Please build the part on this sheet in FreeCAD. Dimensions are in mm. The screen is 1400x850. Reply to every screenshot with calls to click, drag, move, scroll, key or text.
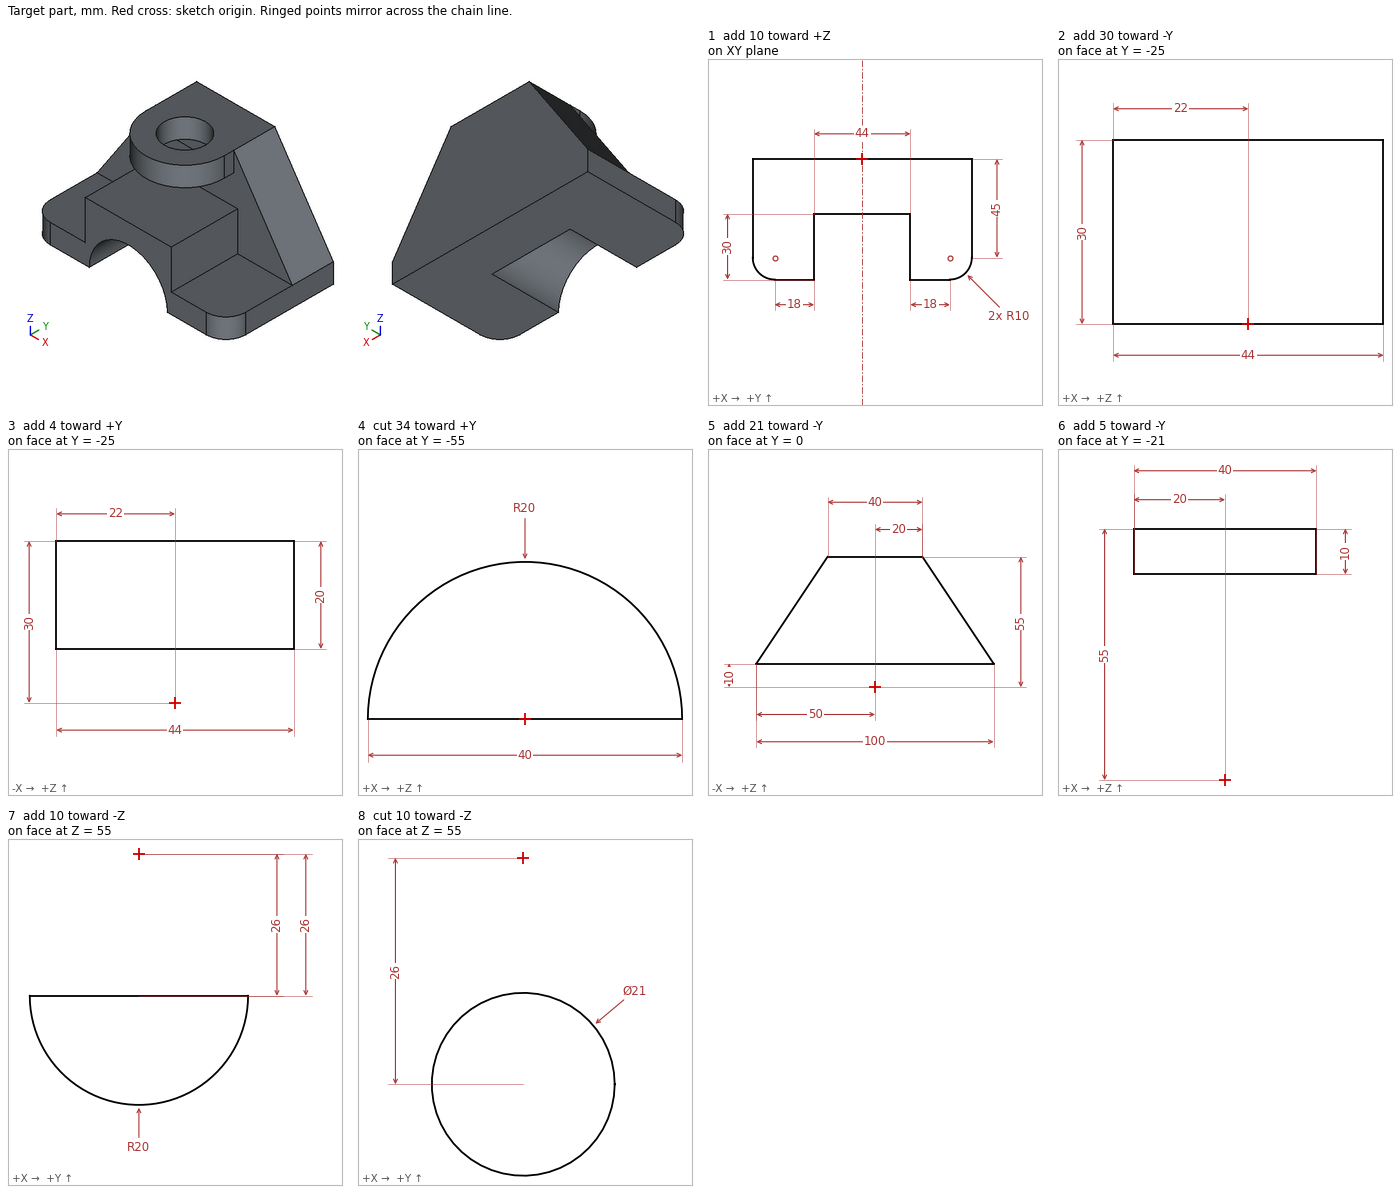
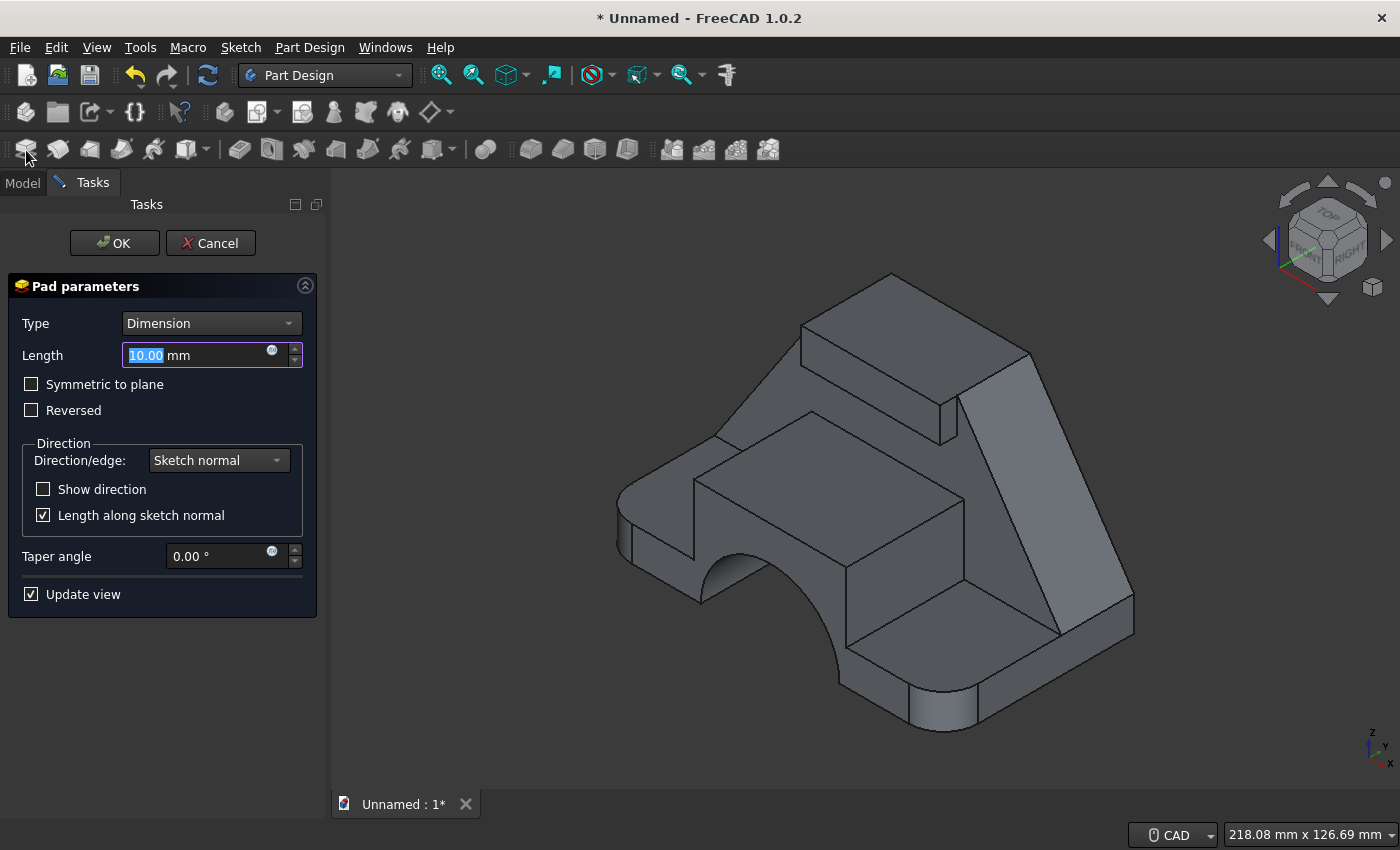
text(10)
key(Tab)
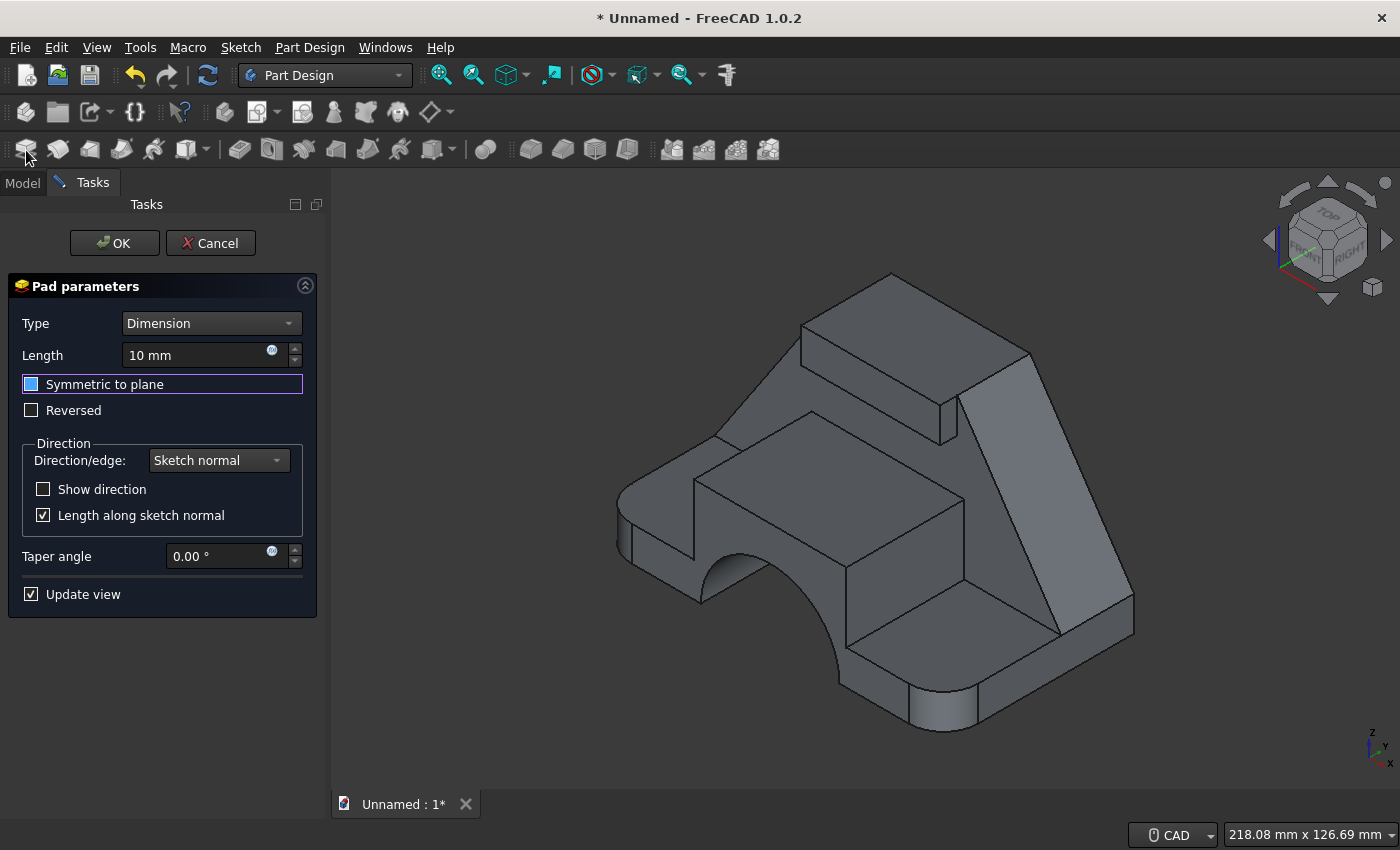
click(30, 410)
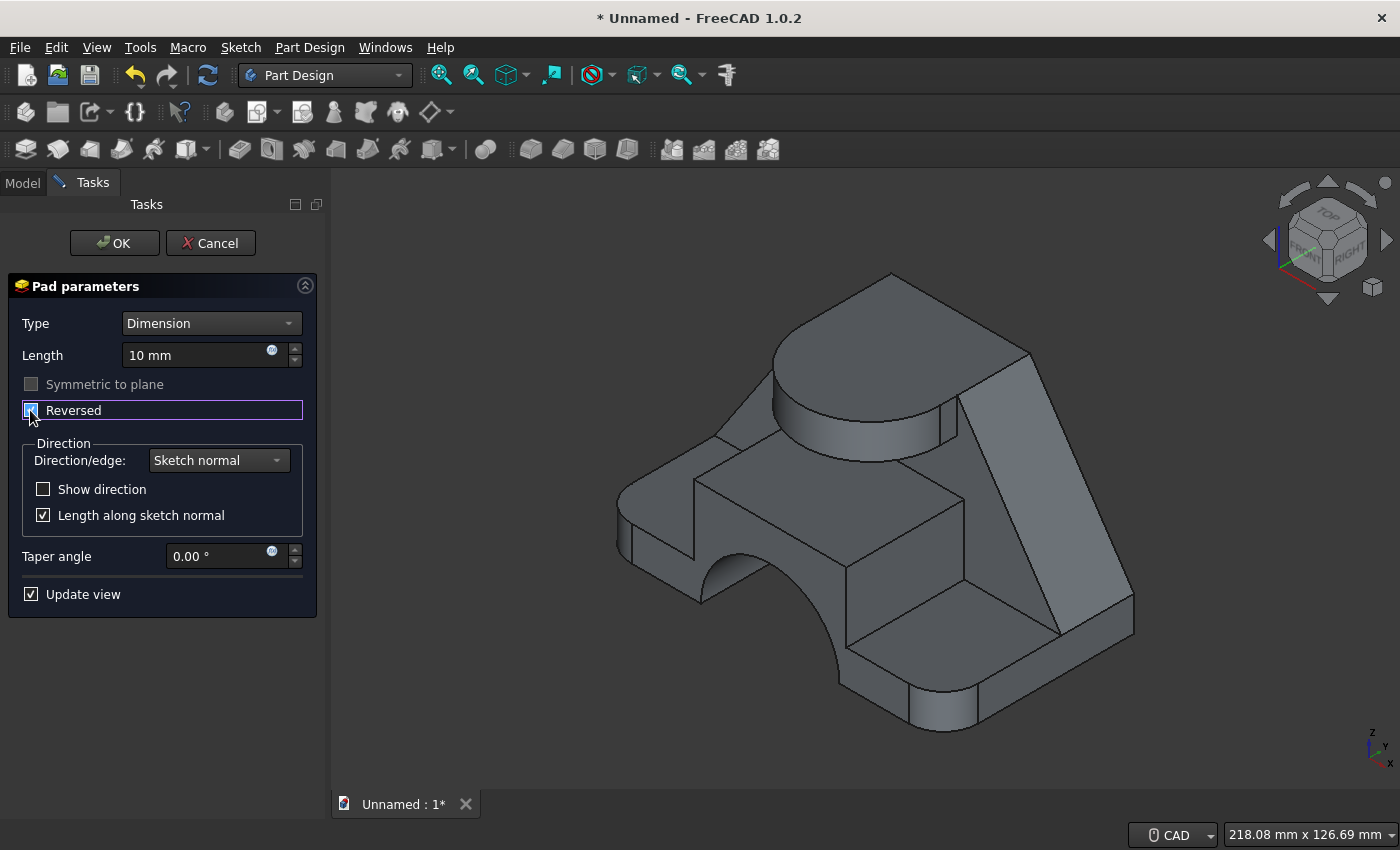
click(115, 243)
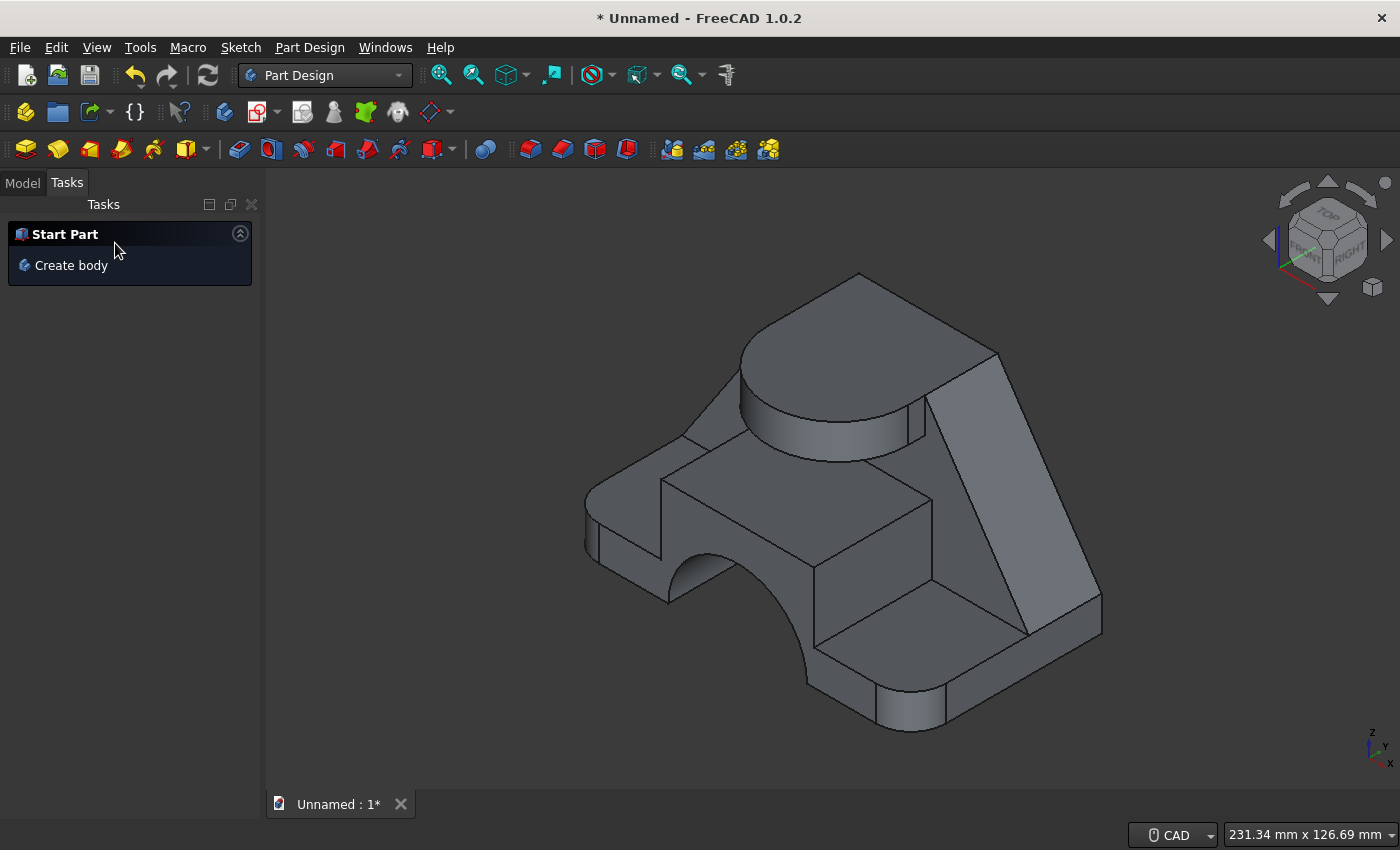
click(849, 358)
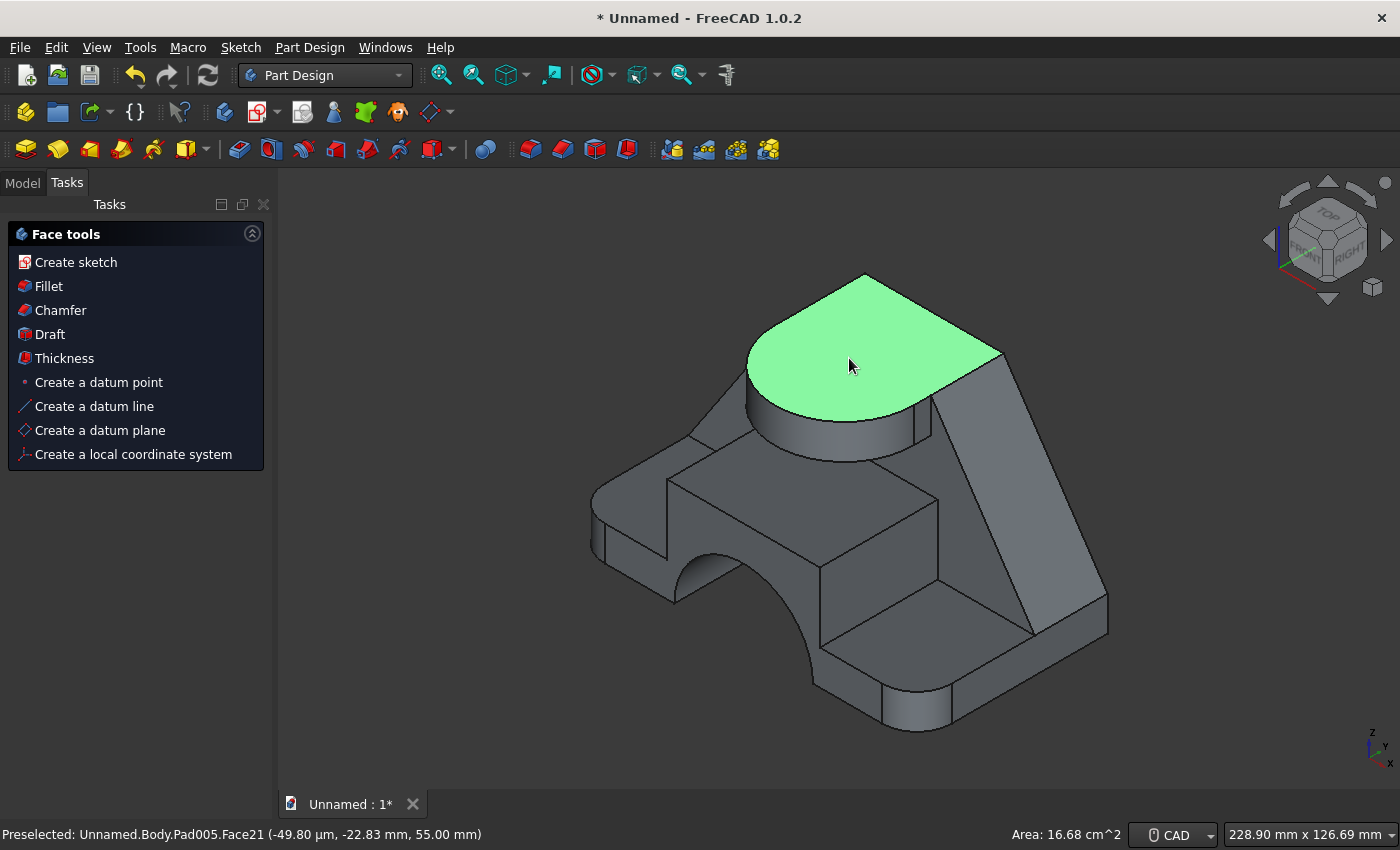
click(258, 112)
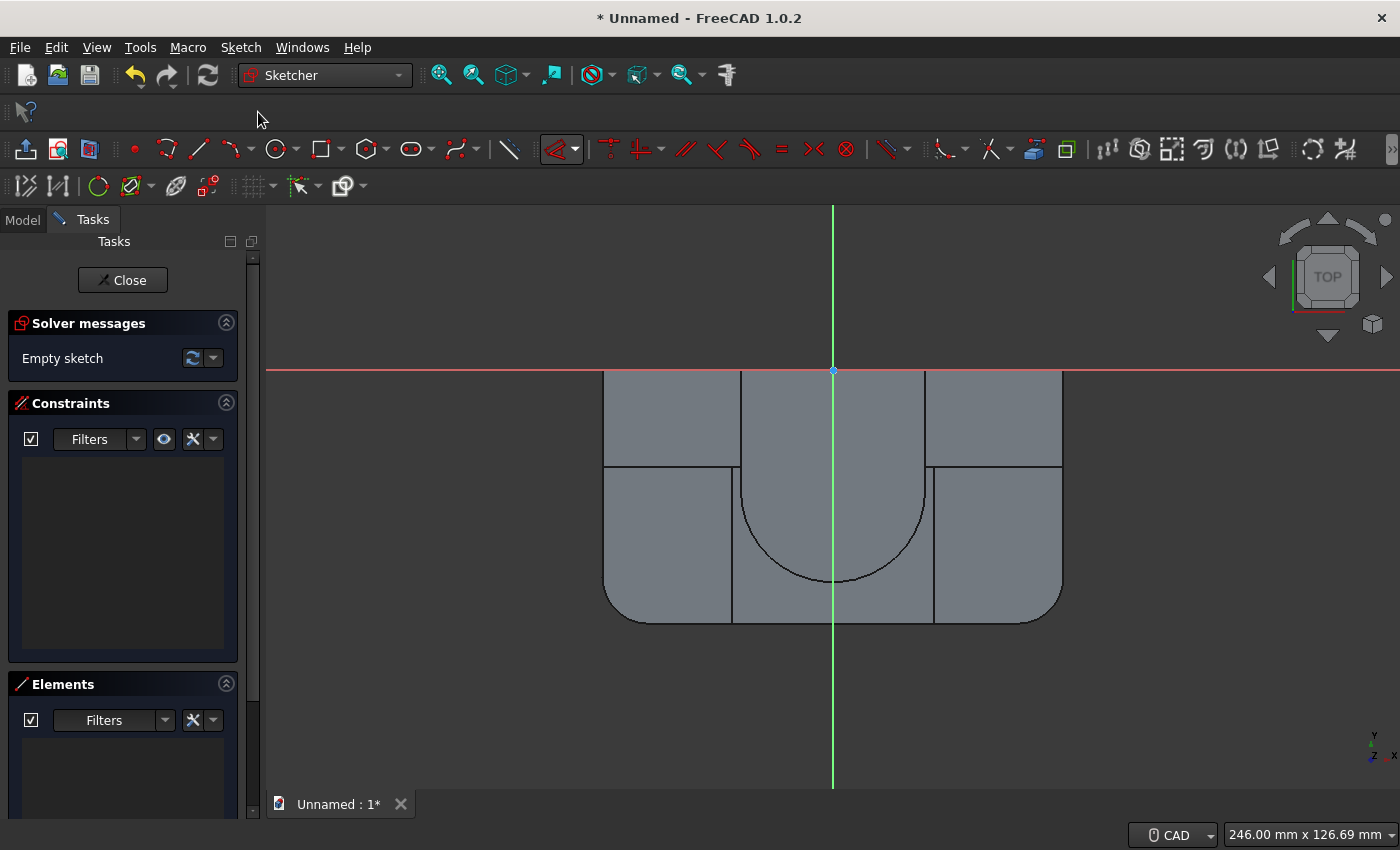
scroll(889, 420, up, 4)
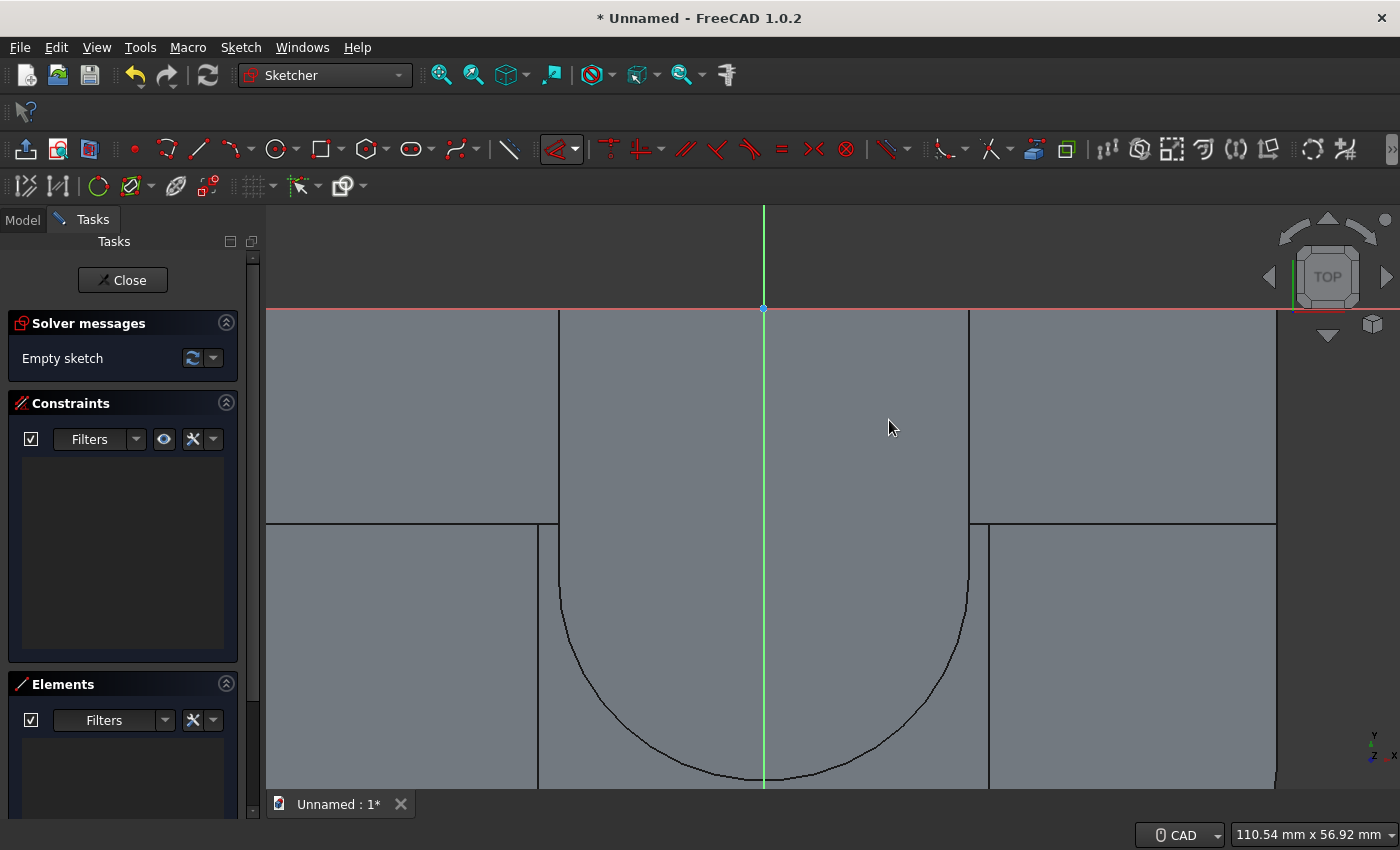
click(276, 150)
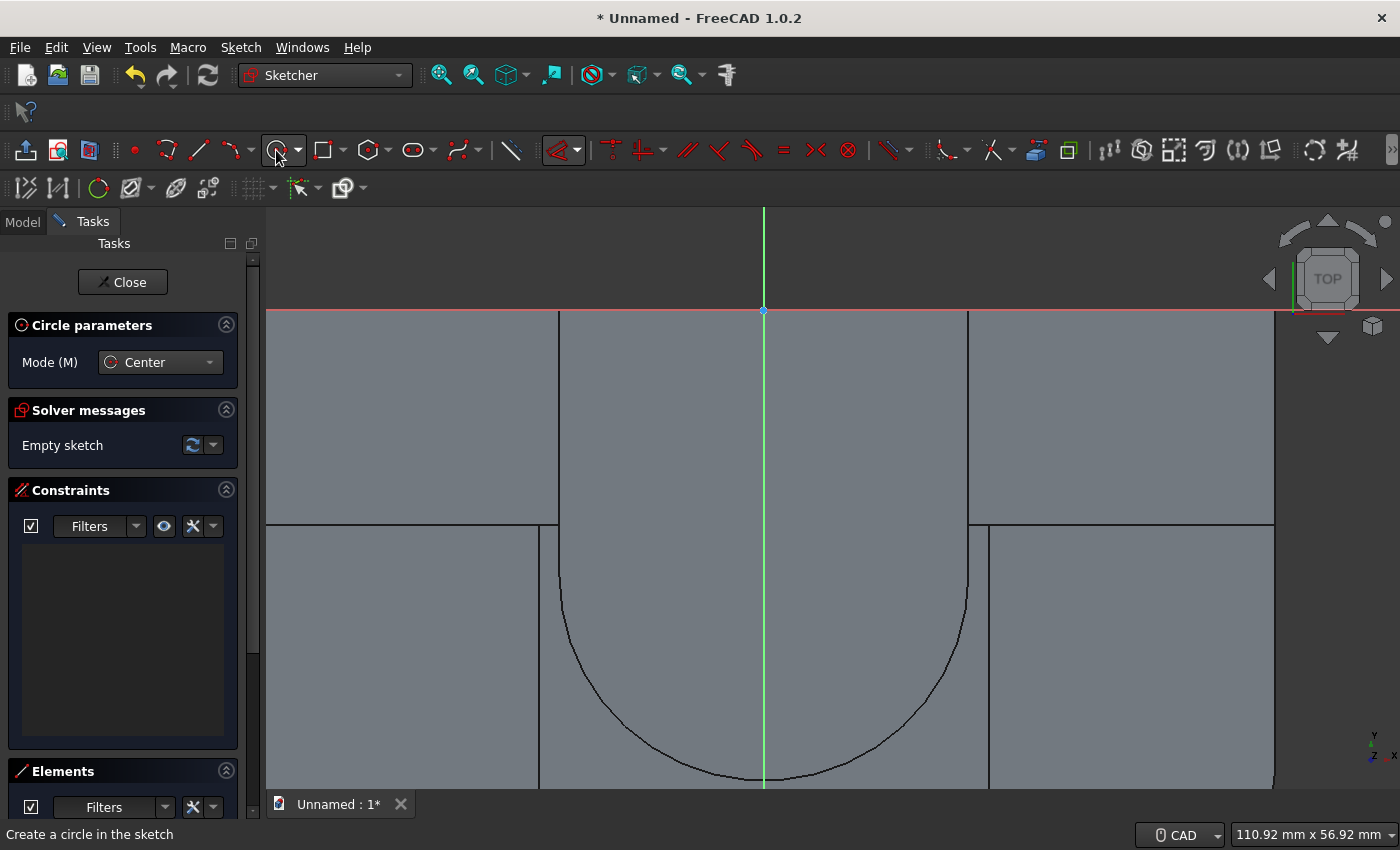
click(764, 576)
move(840, 500)